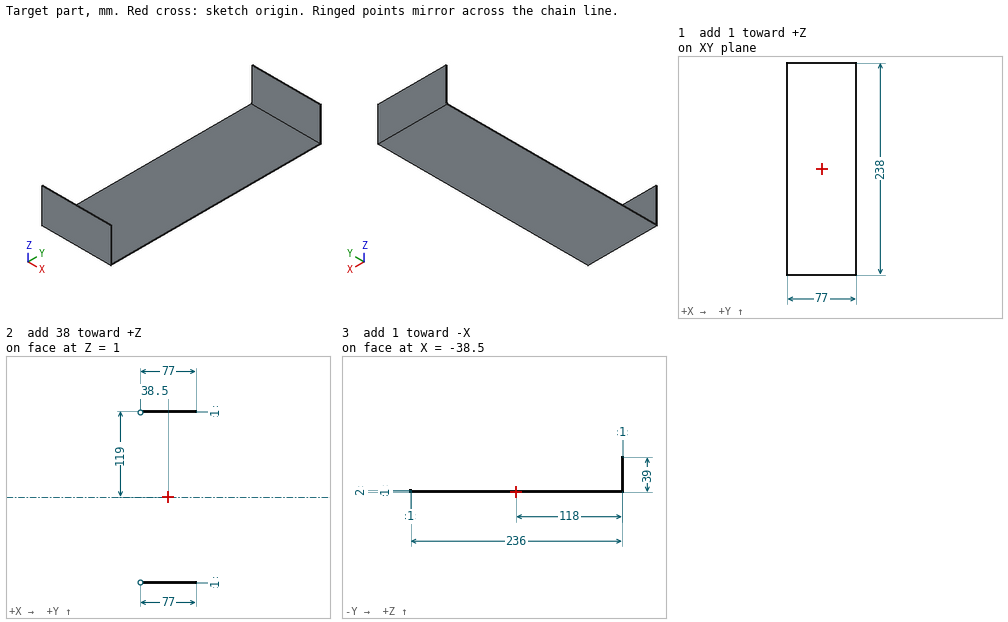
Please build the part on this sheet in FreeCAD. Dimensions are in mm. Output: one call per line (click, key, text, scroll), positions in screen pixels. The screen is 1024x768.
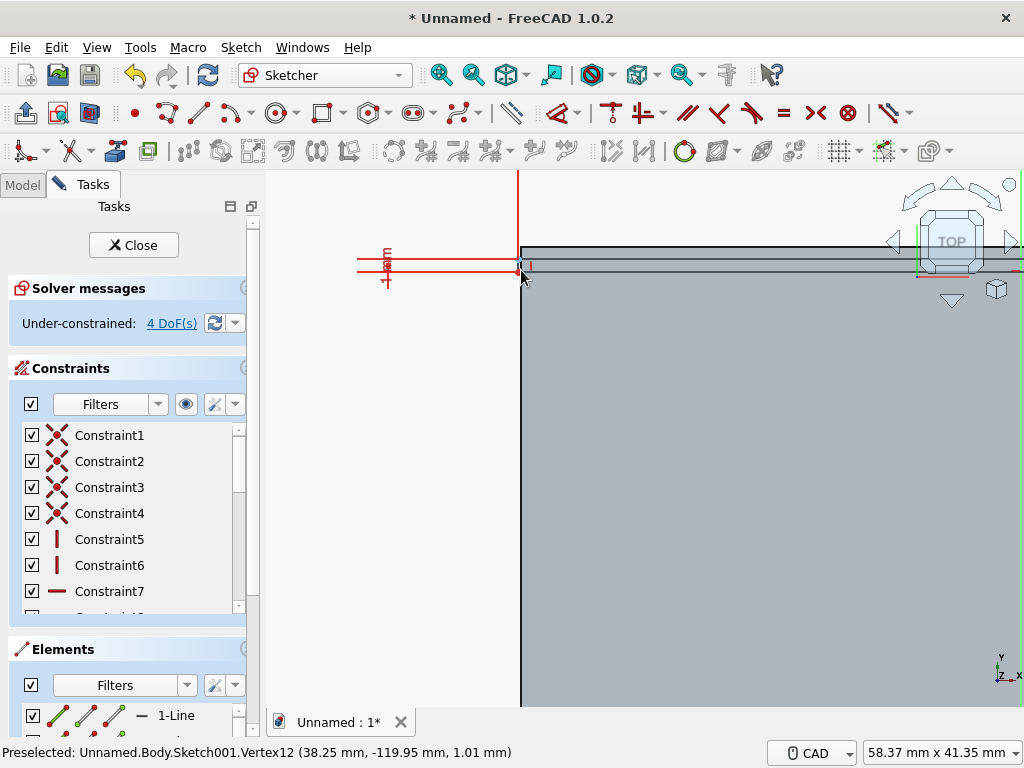
click(518, 272)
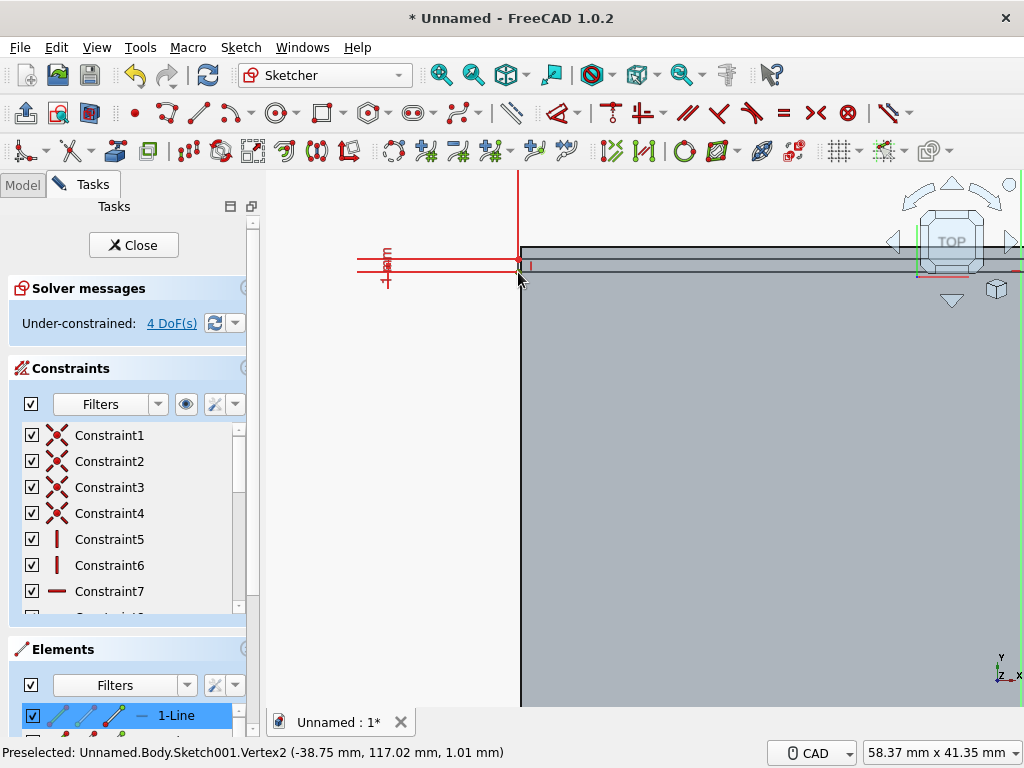
scroll(521, 270, down, 11)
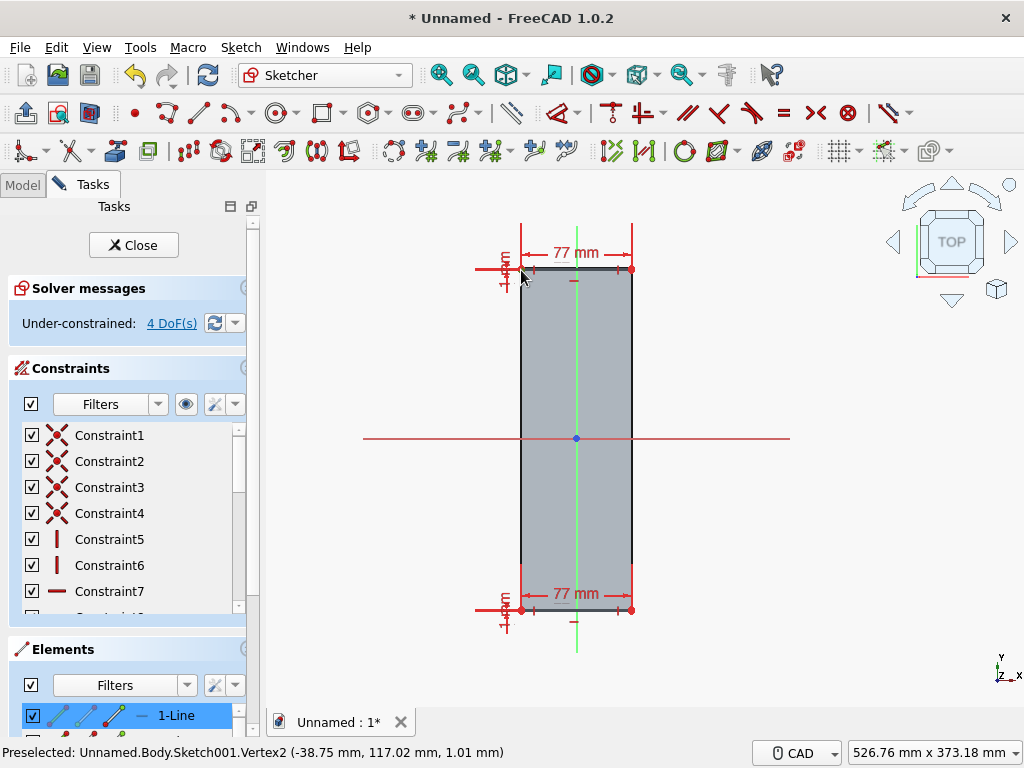
scroll(521, 610, up, 11)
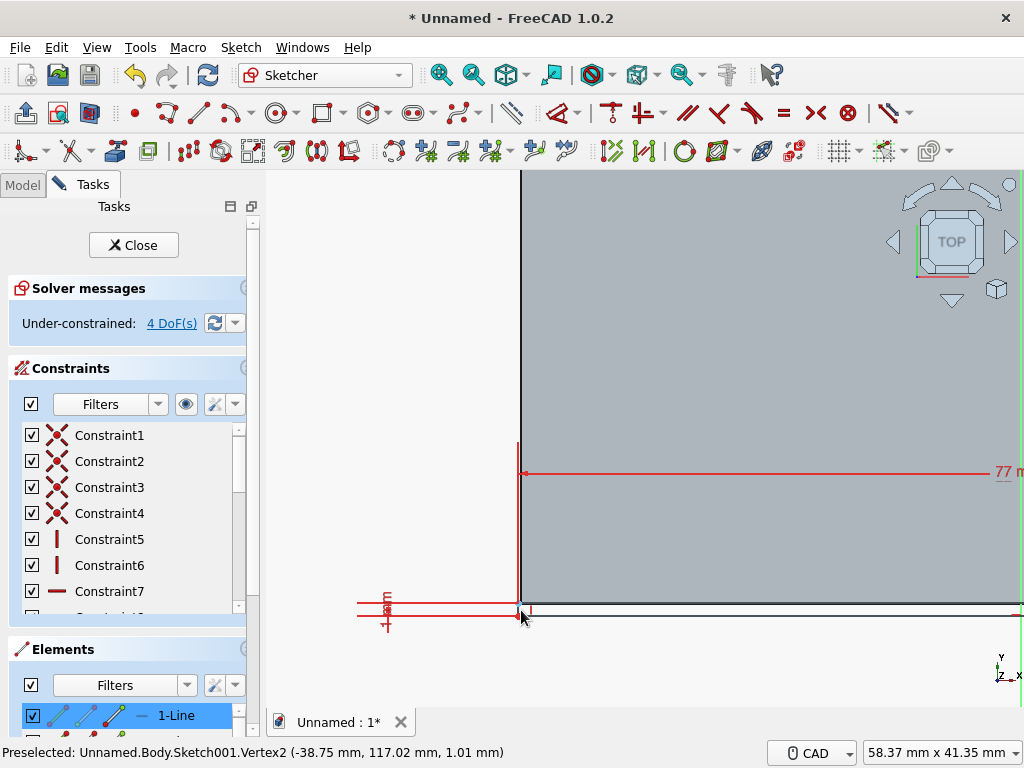
click(518, 603)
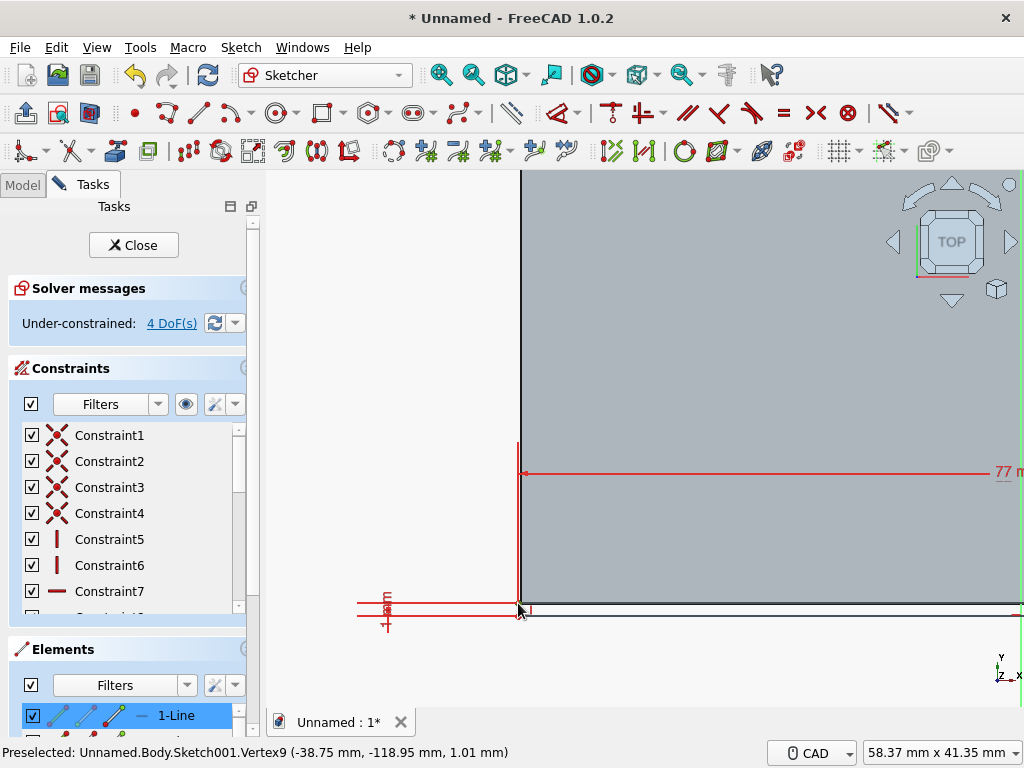
scroll(521, 610, down, 11)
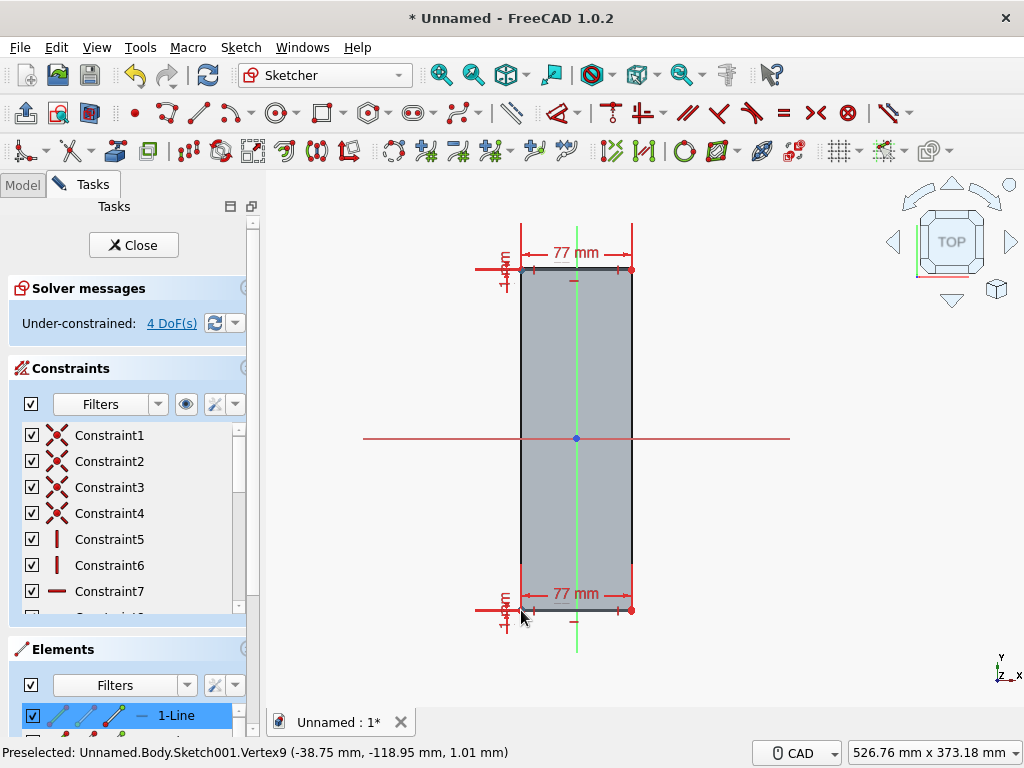
click(375, 439)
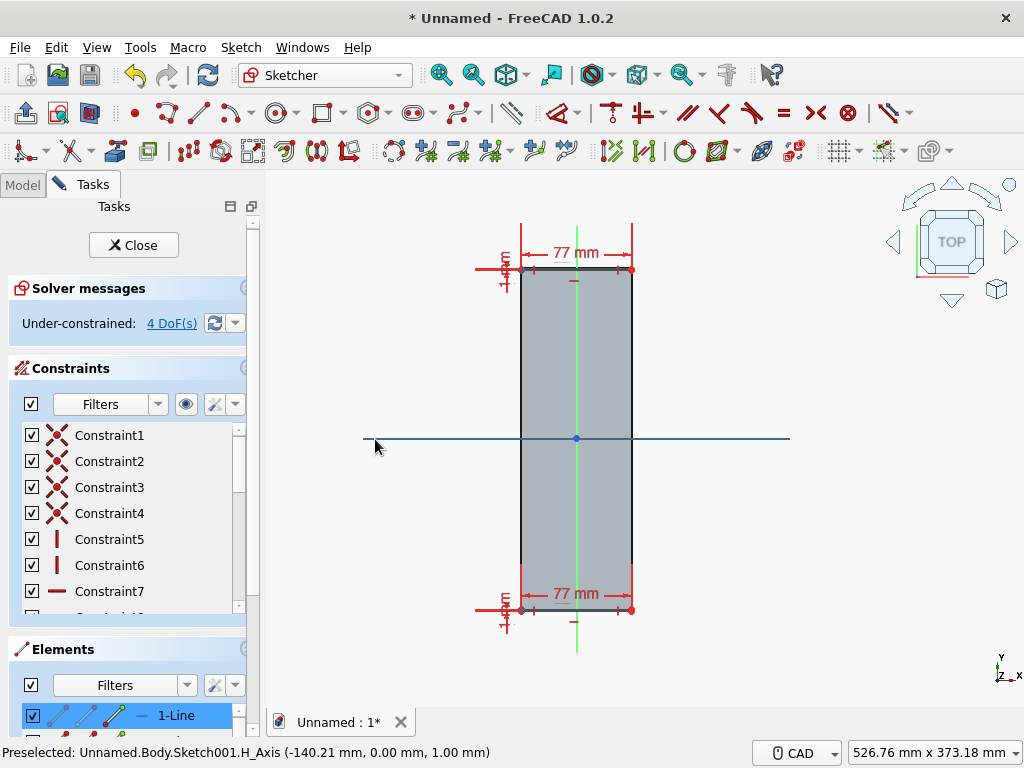
click(816, 114)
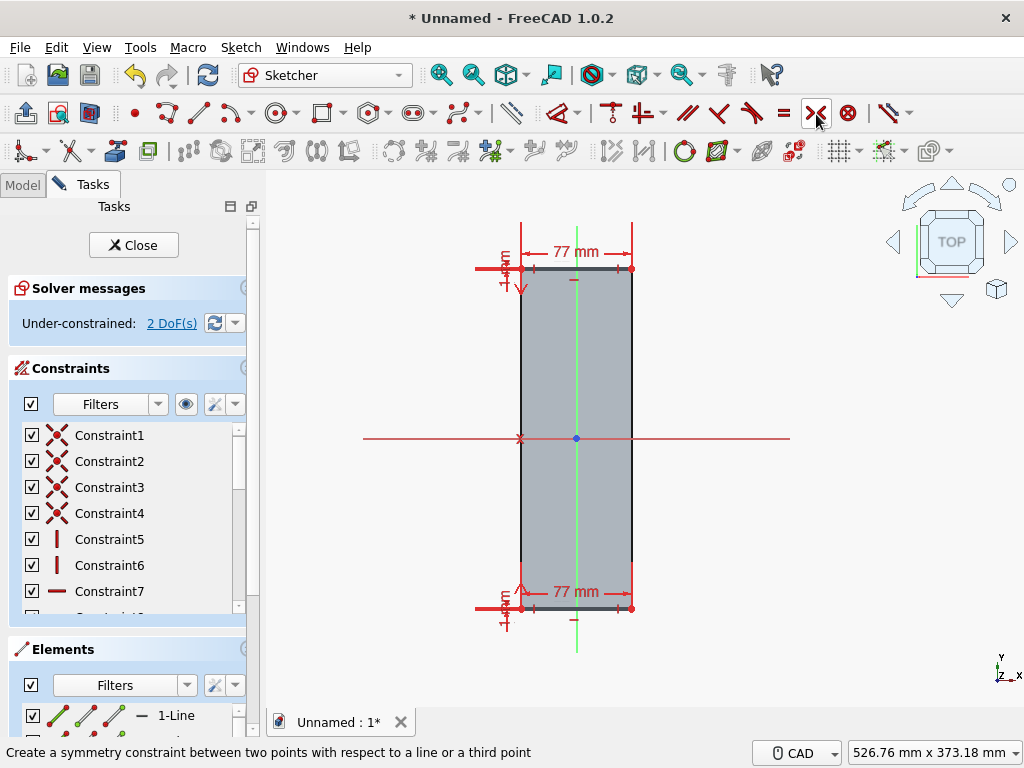
click(558, 114)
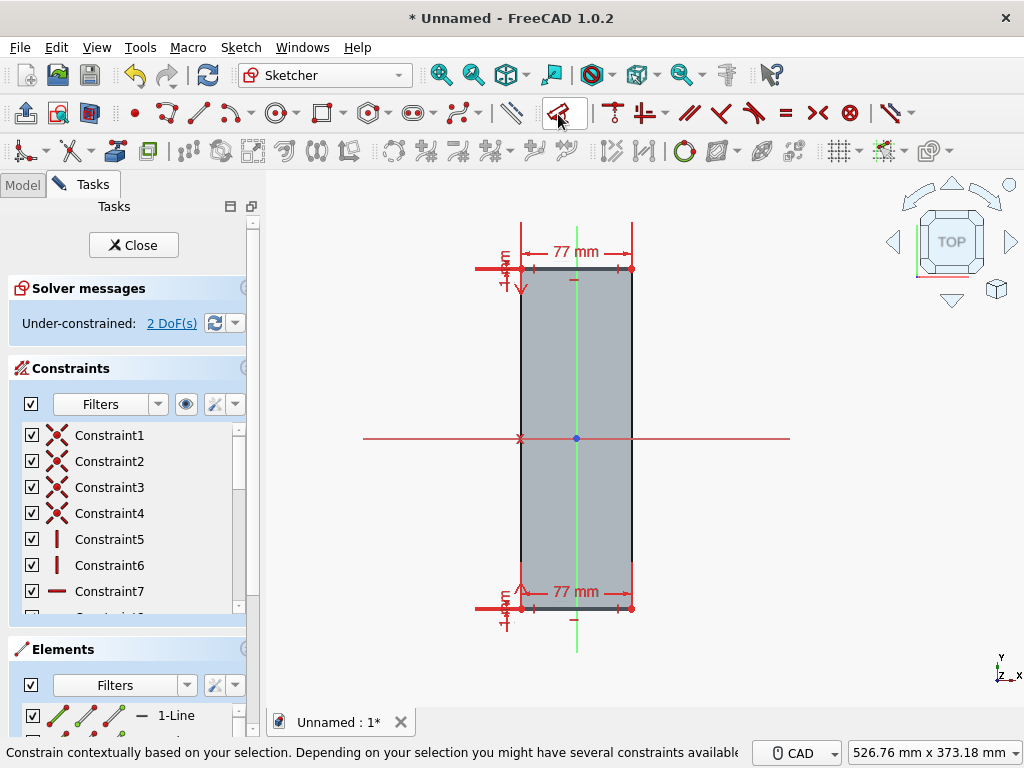
scroll(521, 268, up, 11)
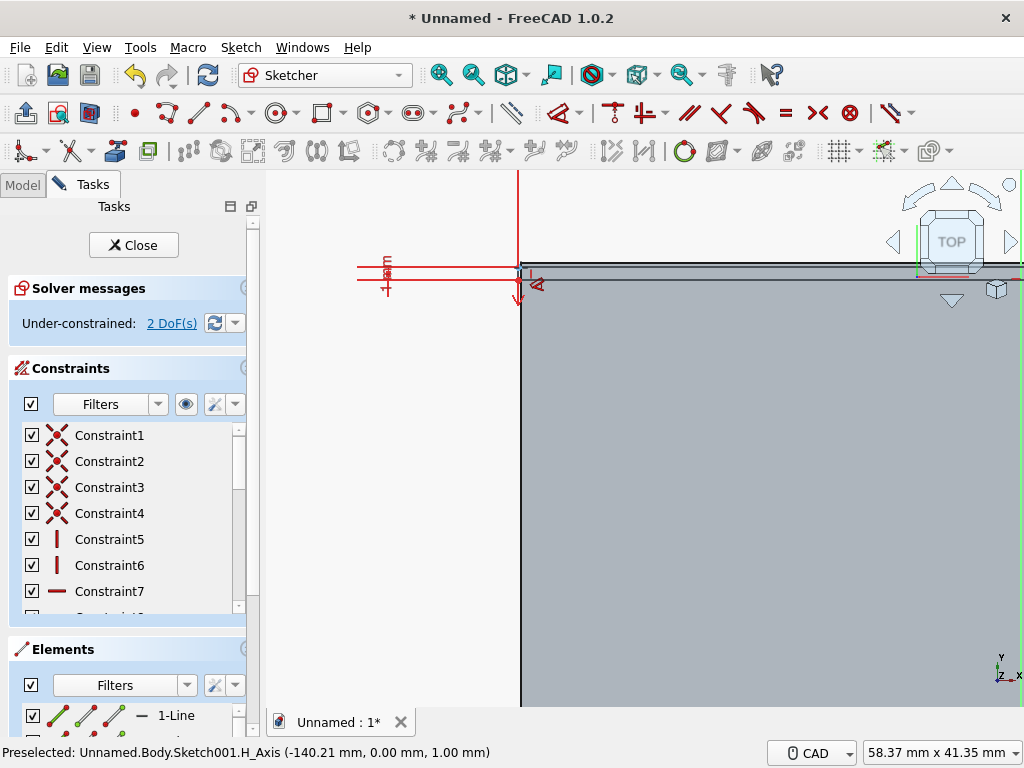
click(518, 267)
click(484, 473)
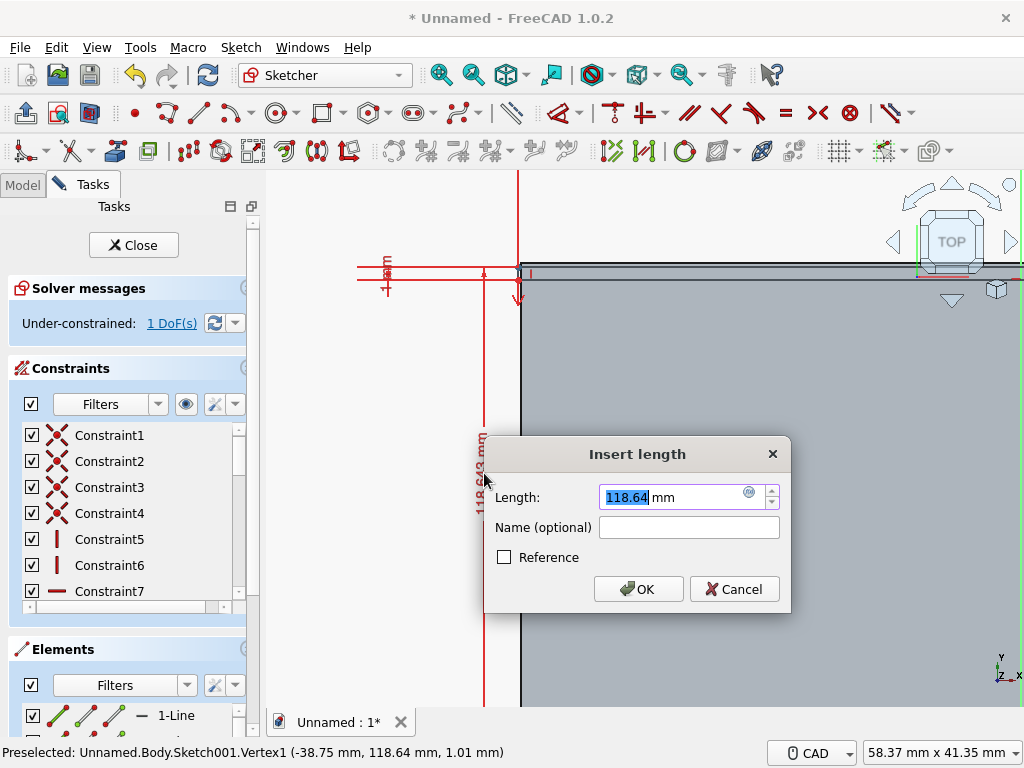
text(119)
key(Return)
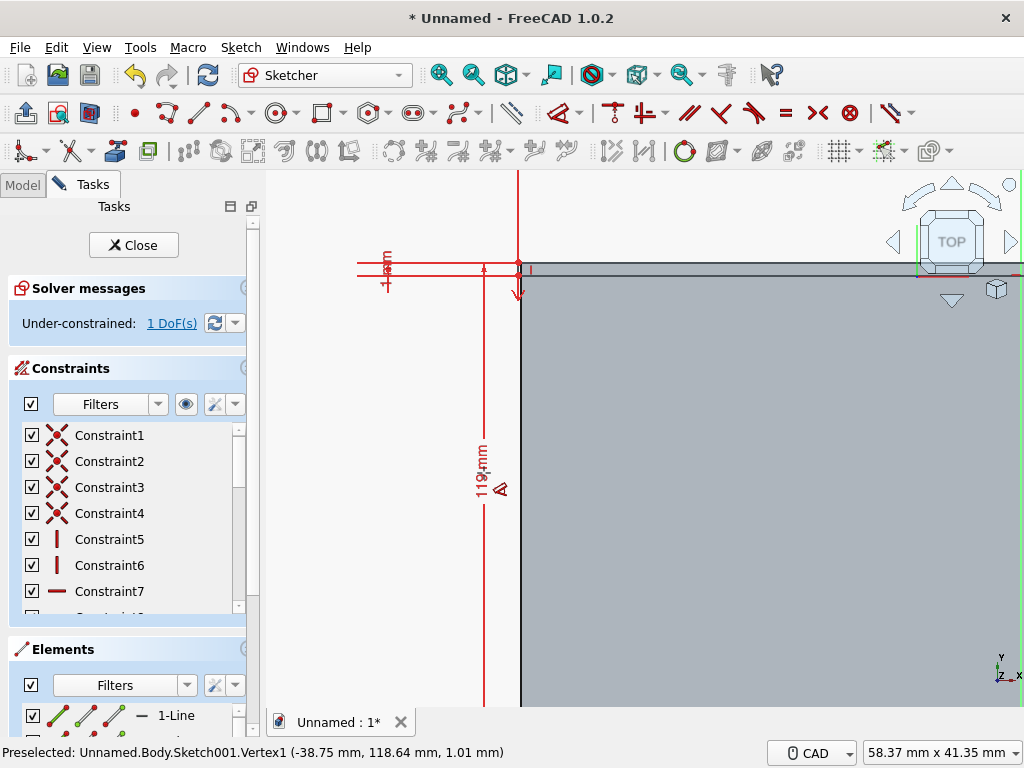
click(518, 263)
click(689, 229)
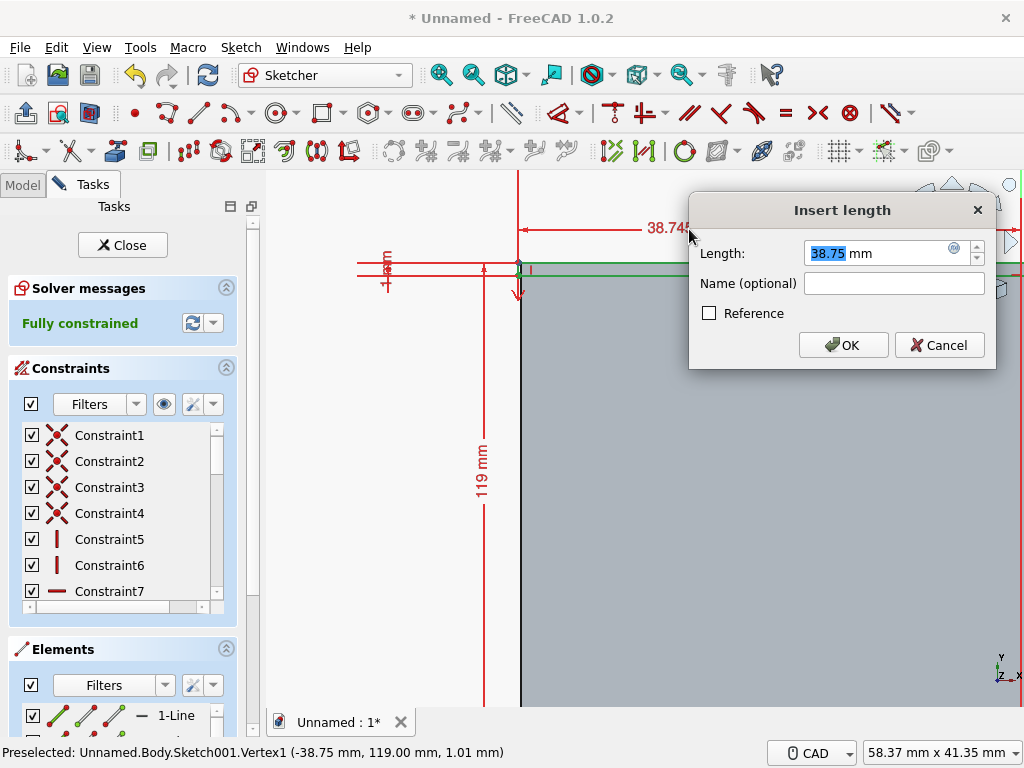
text(38.5)
key(Return)
key(Escape)